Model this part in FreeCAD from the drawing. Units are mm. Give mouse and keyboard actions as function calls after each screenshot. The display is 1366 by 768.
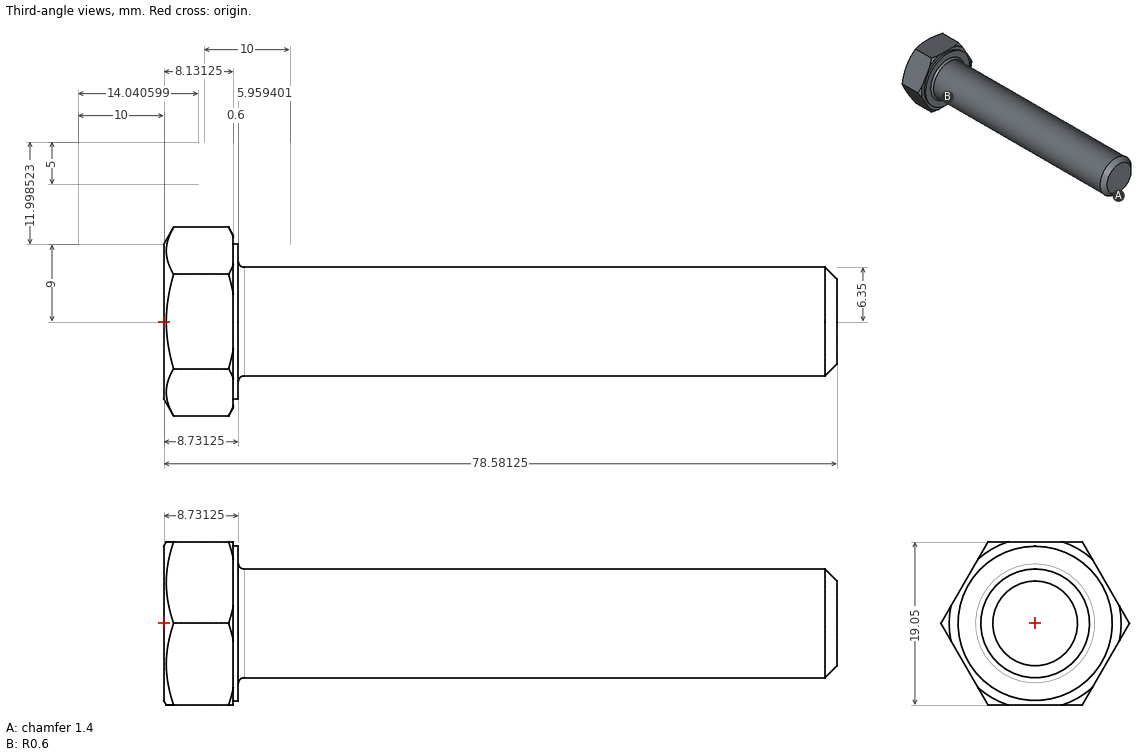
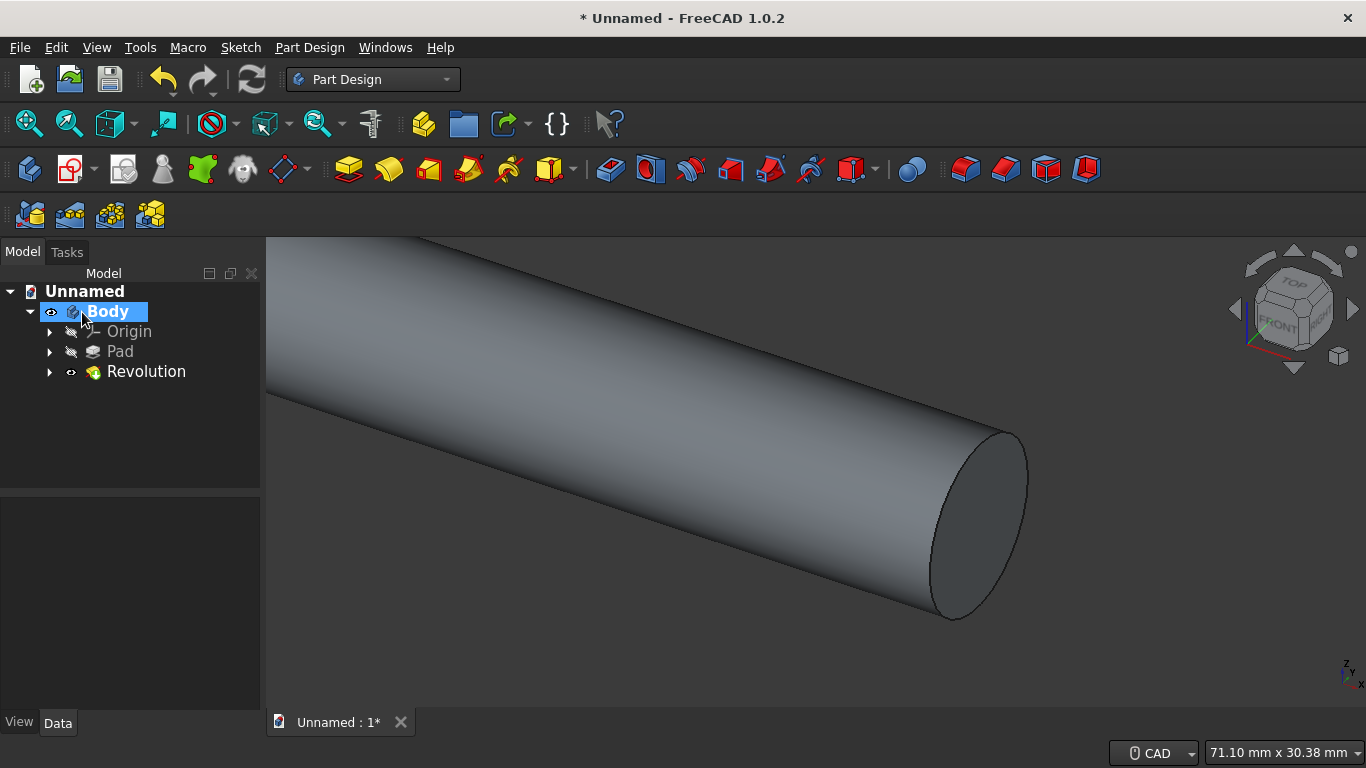
click(30, 124)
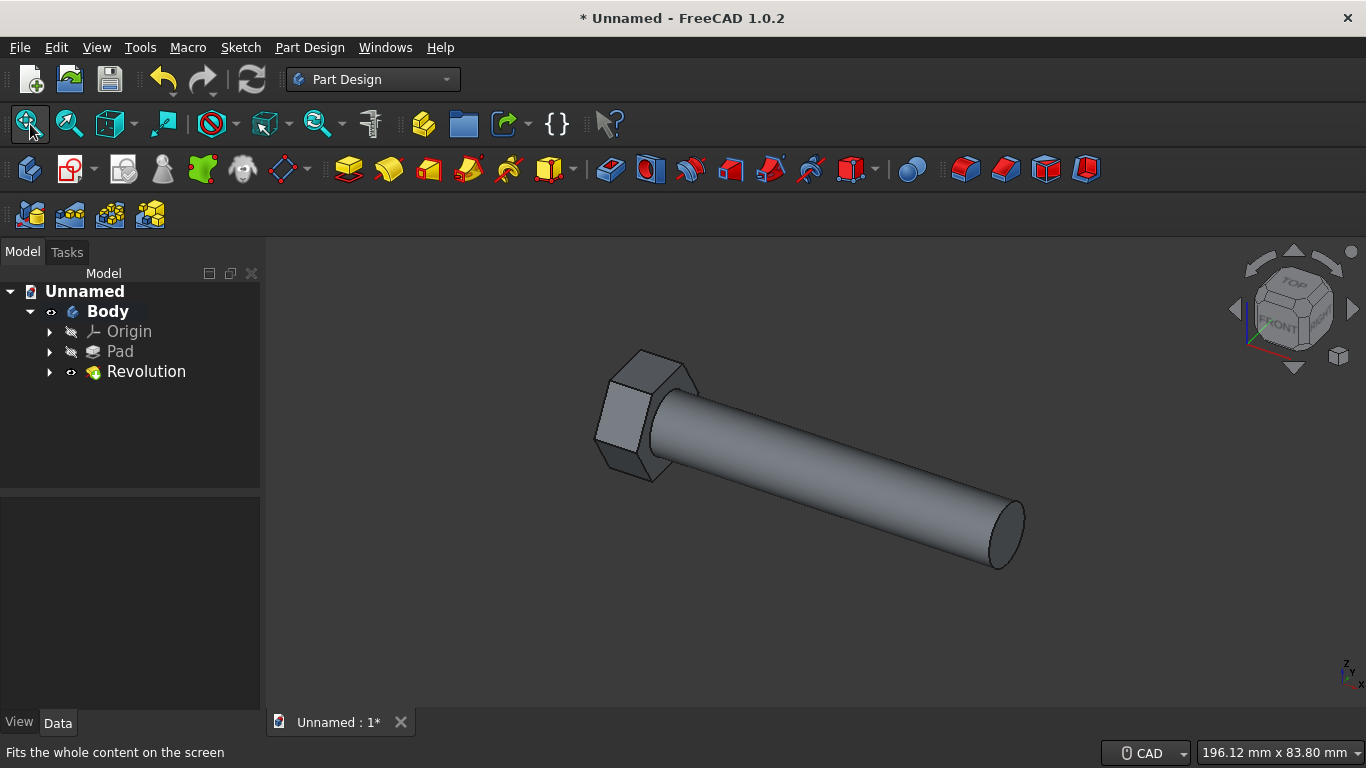
click(70, 170)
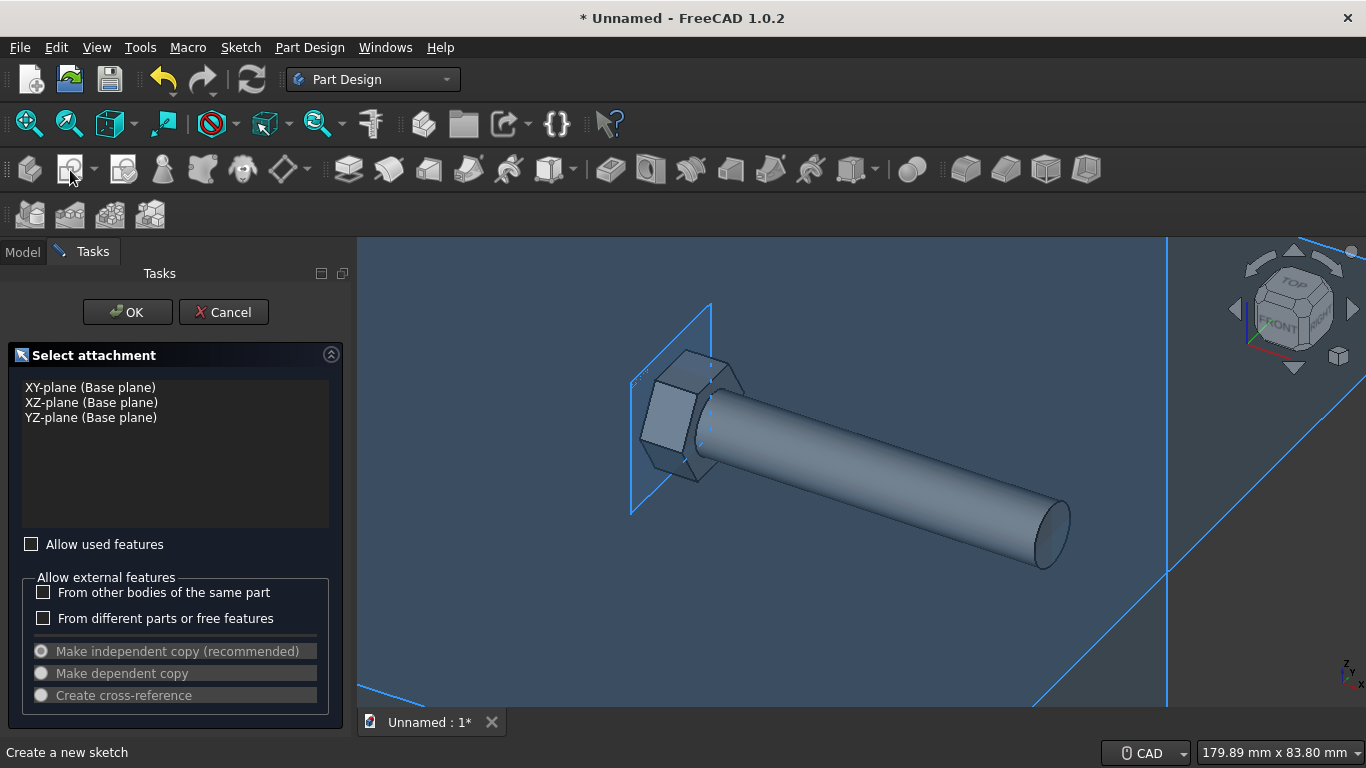
click(82, 388)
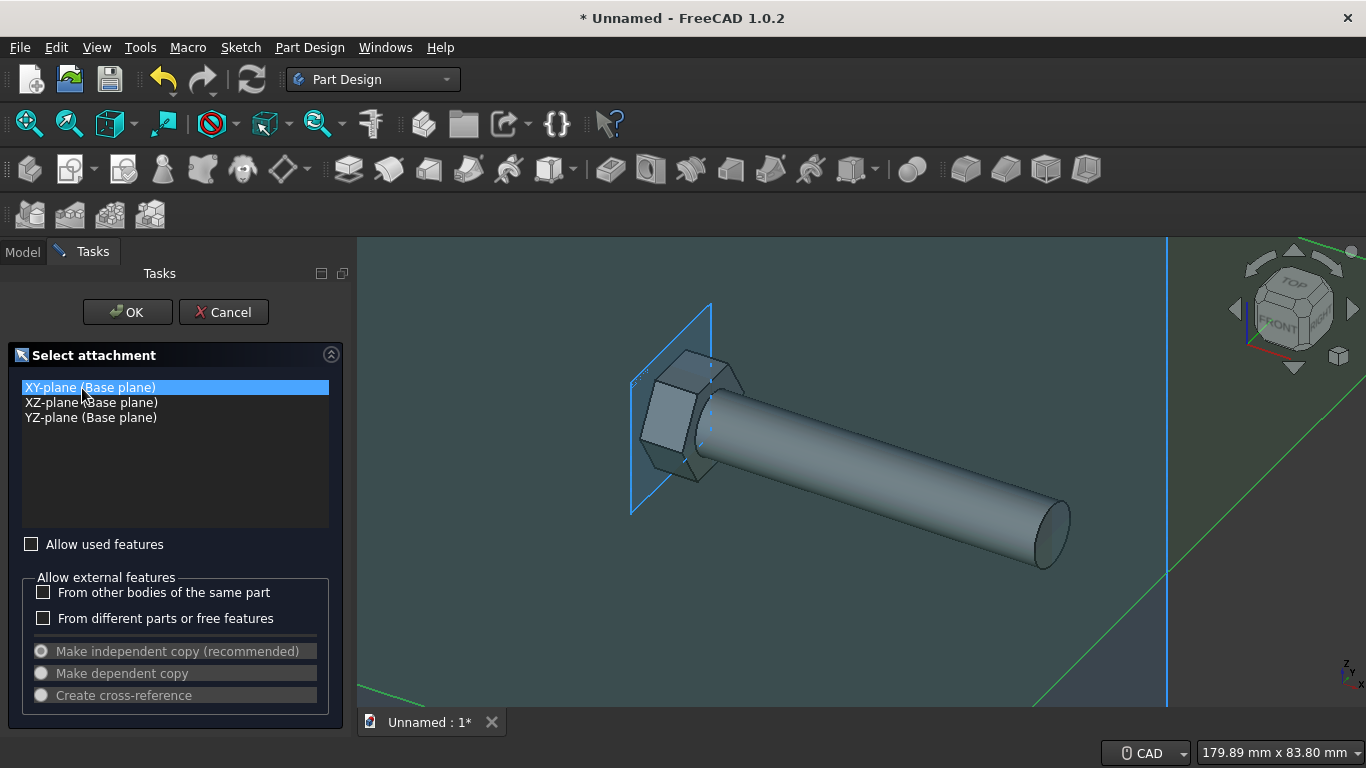
click(128, 312)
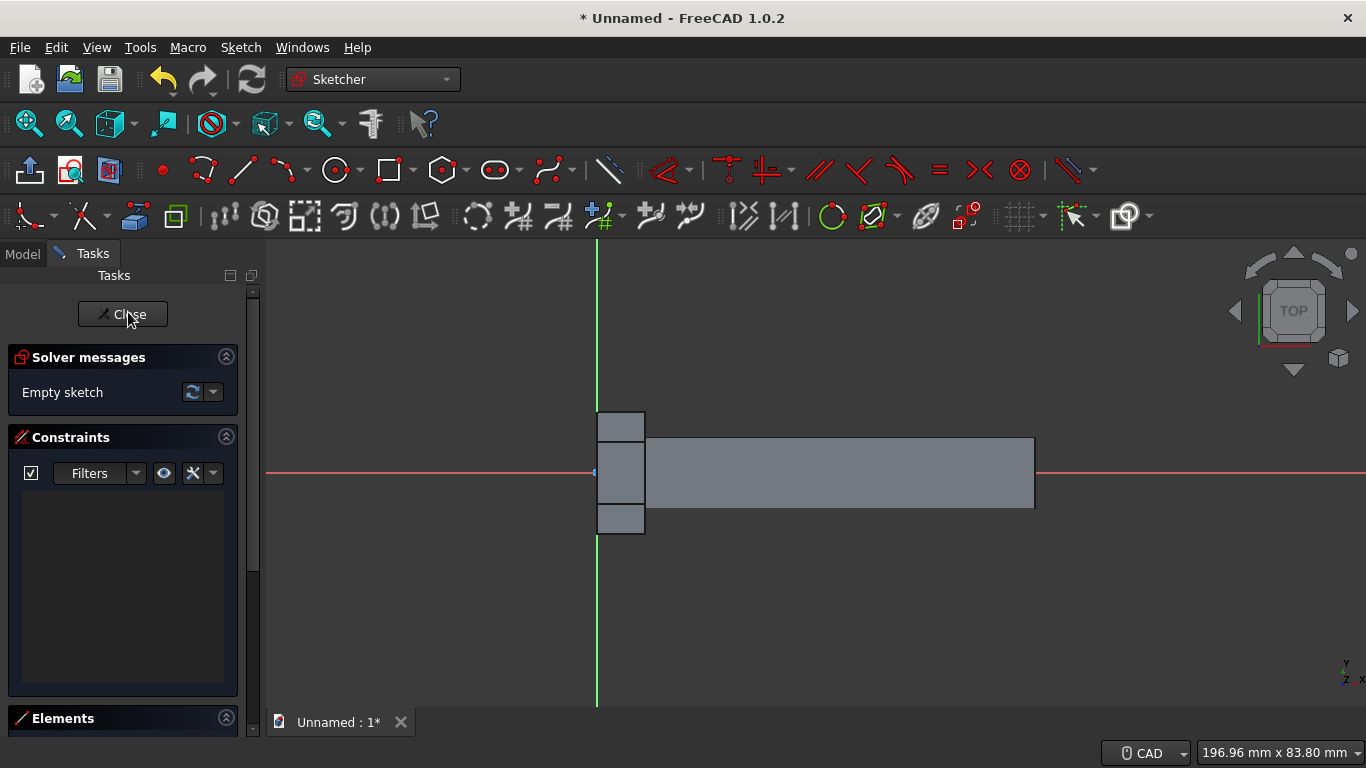
click(110, 170)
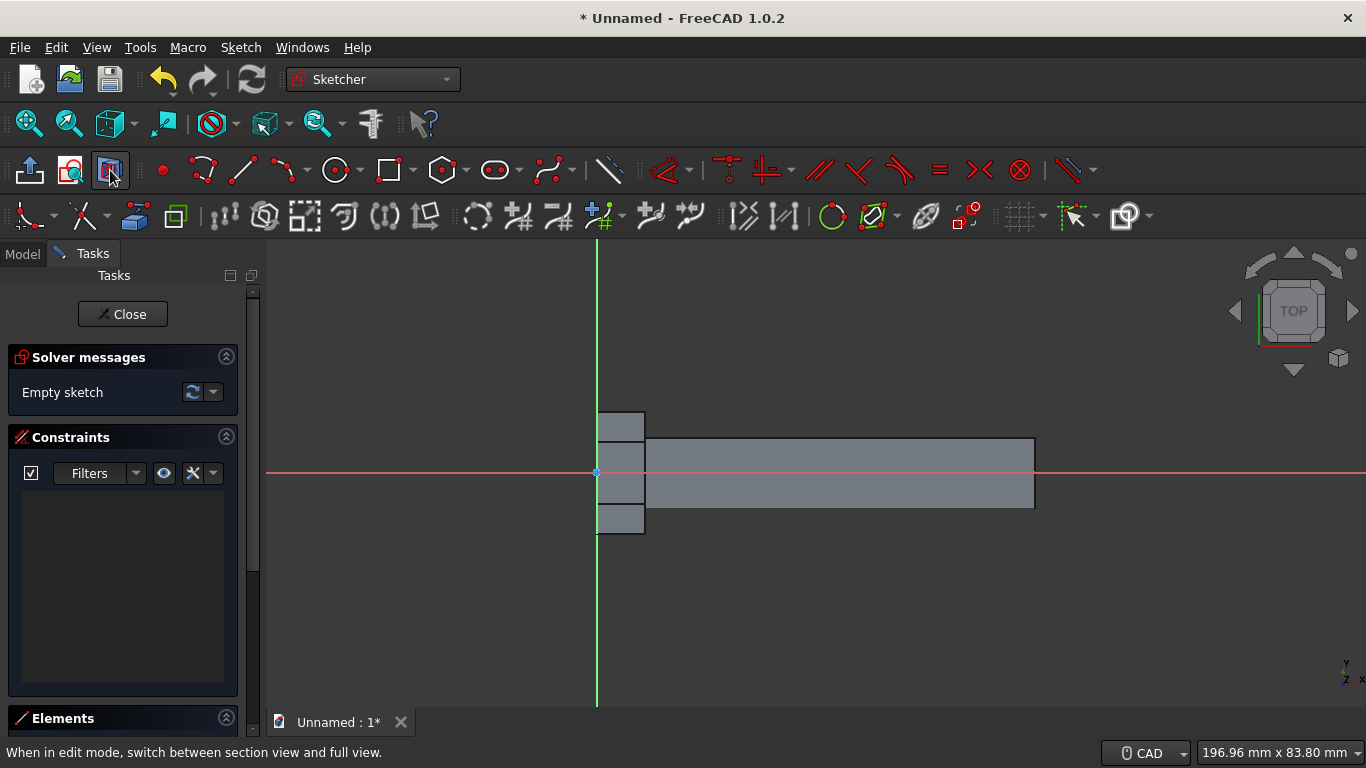
scroll(482, 380, up, 5)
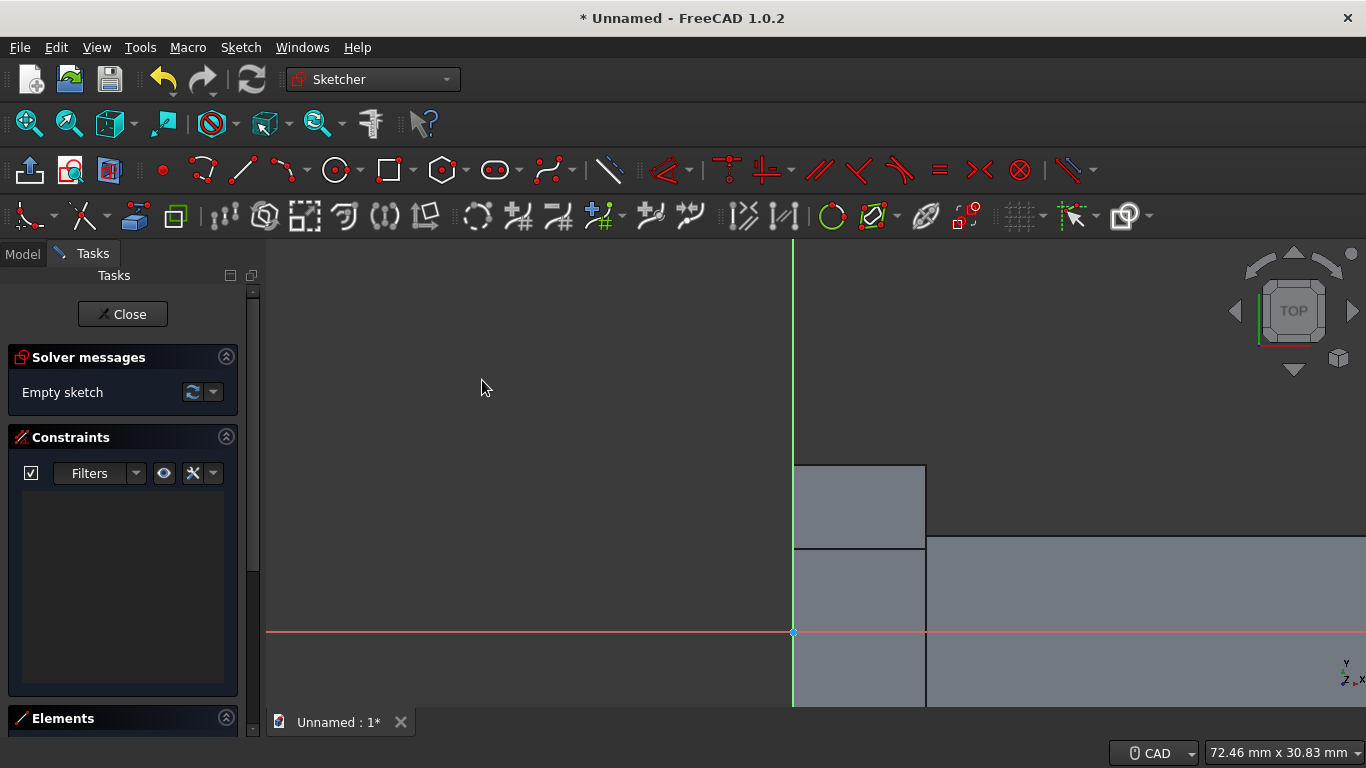
click(204, 170)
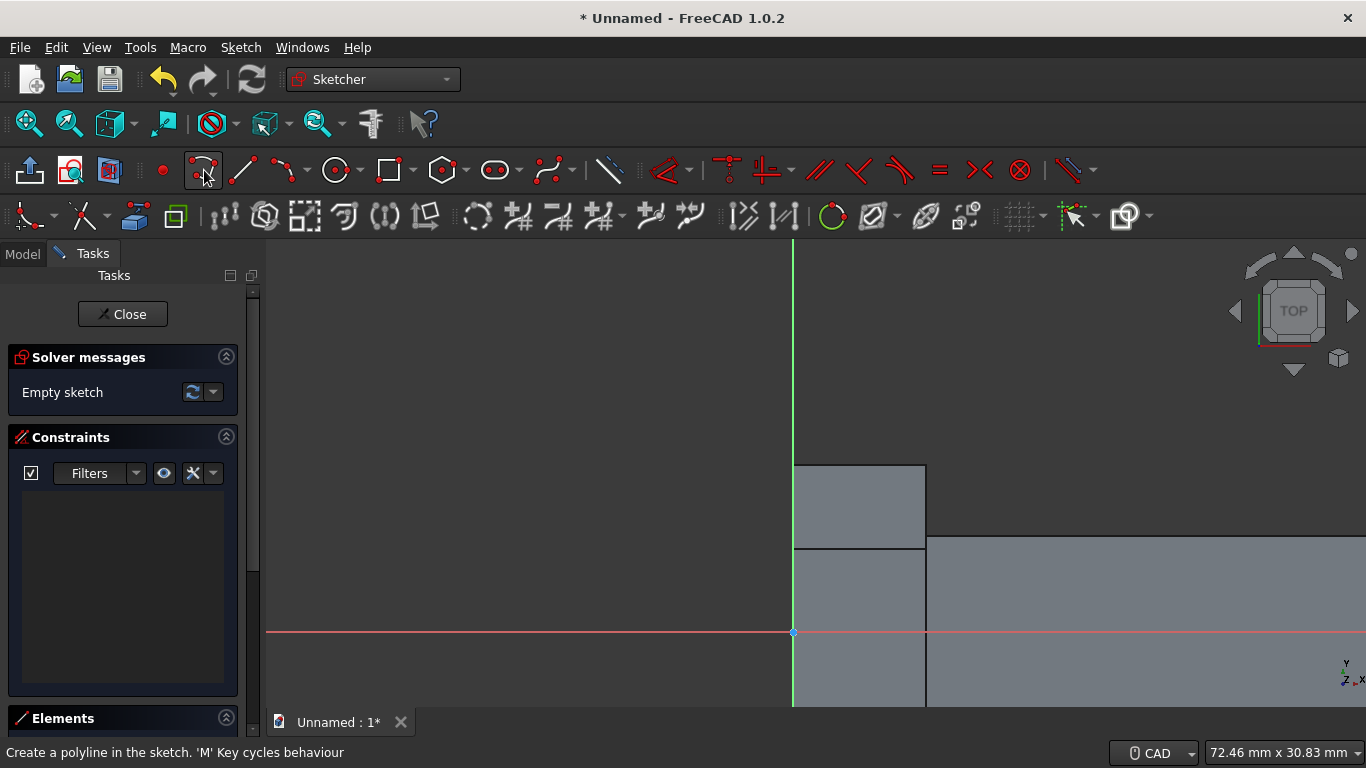
click(793, 496)
click(854, 389)
click(854, 313)
click(641, 313)
click(641, 496)
click(793, 497)
key(Escape)
key(Escape)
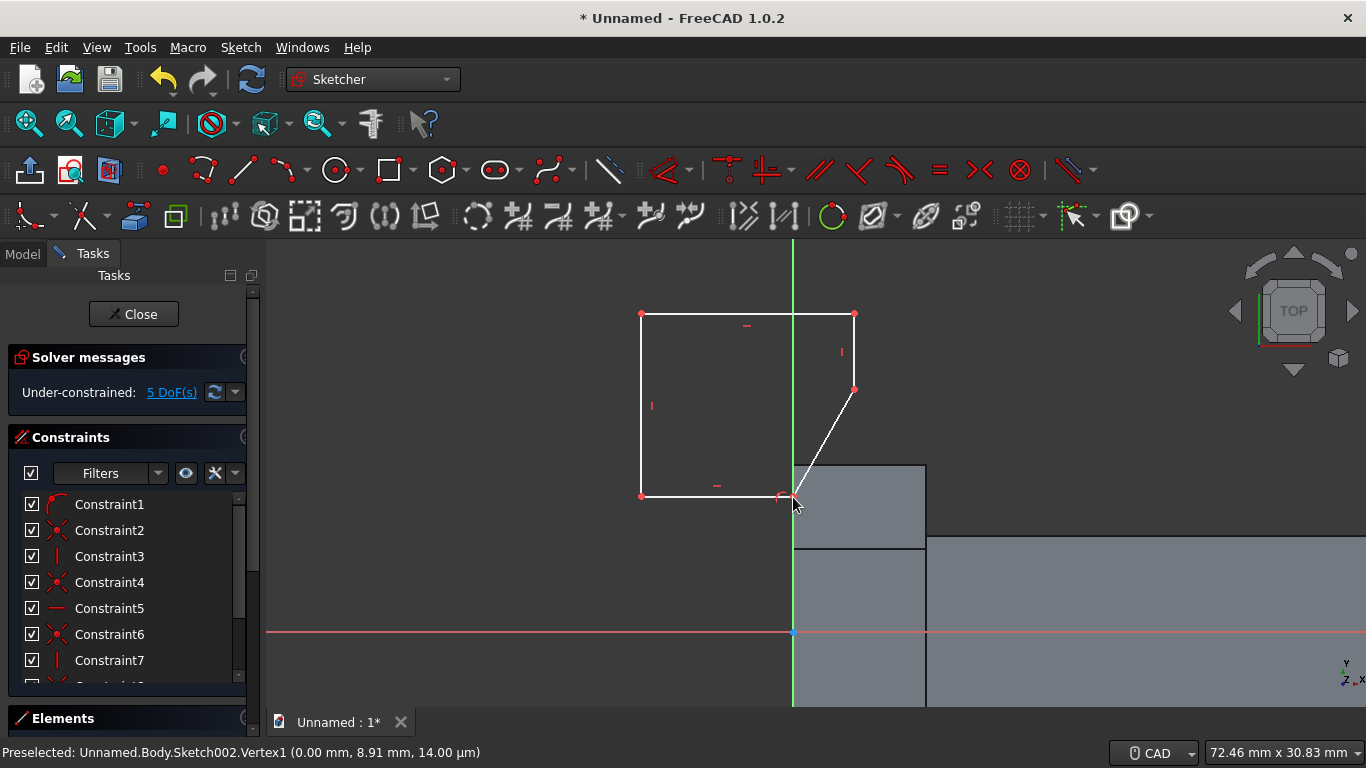
click(664, 170)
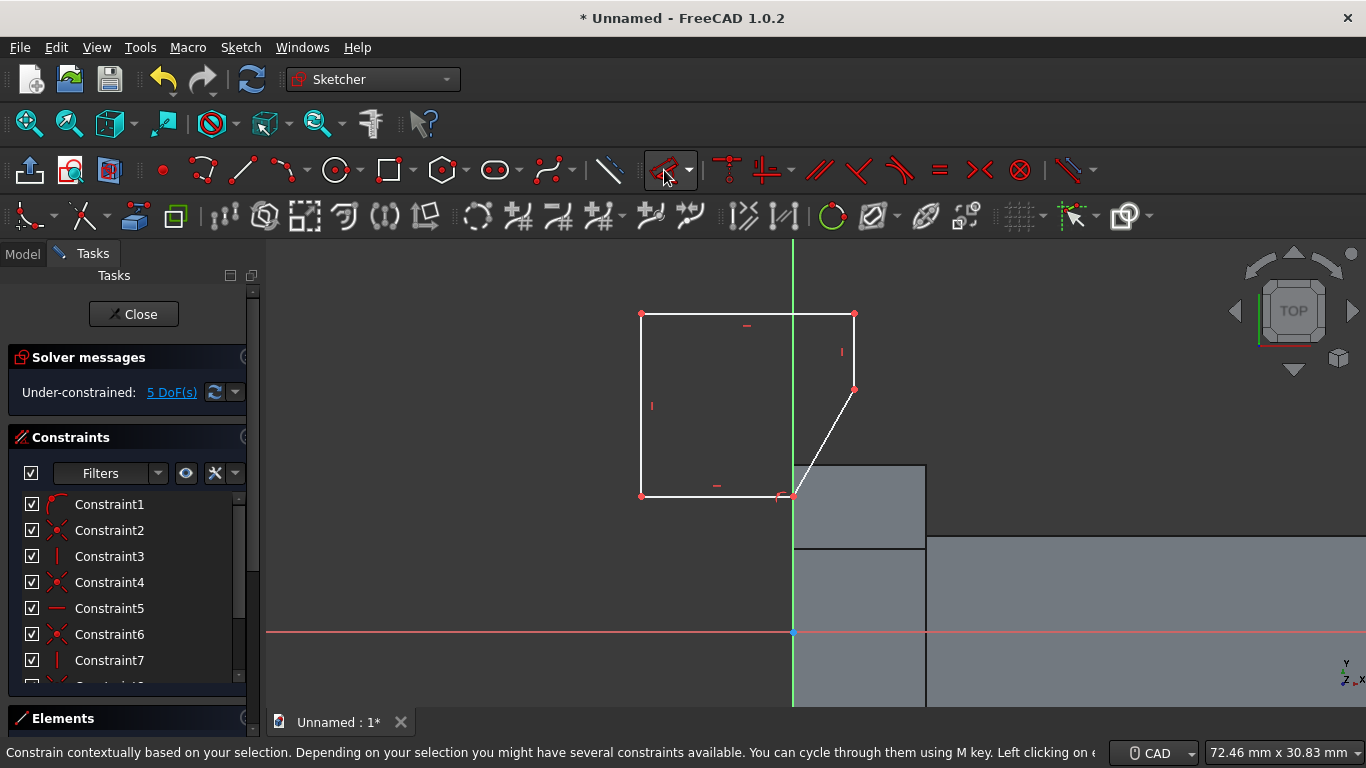
click(854, 367)
click(888, 352)